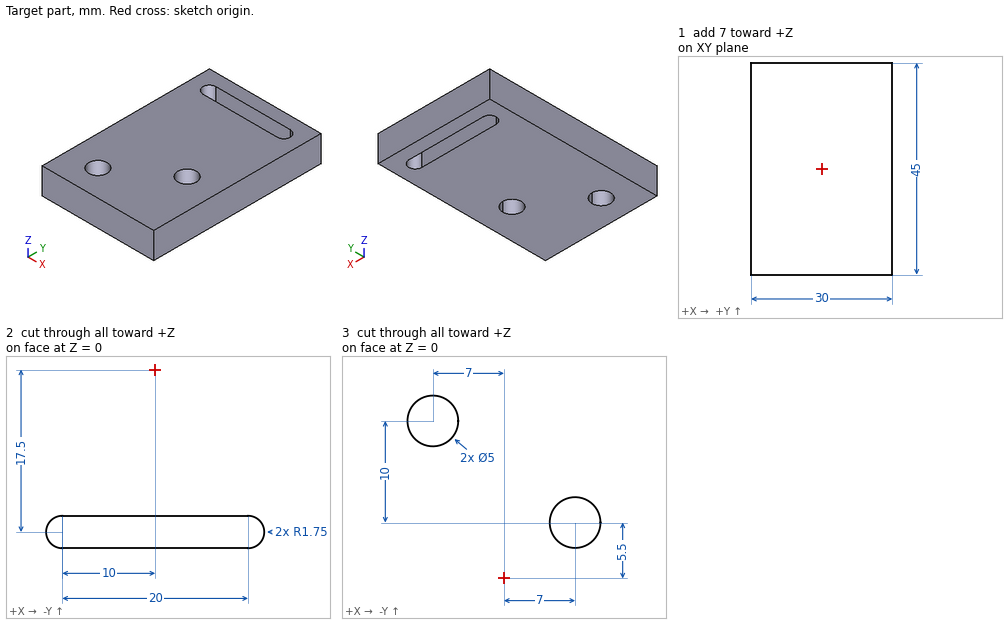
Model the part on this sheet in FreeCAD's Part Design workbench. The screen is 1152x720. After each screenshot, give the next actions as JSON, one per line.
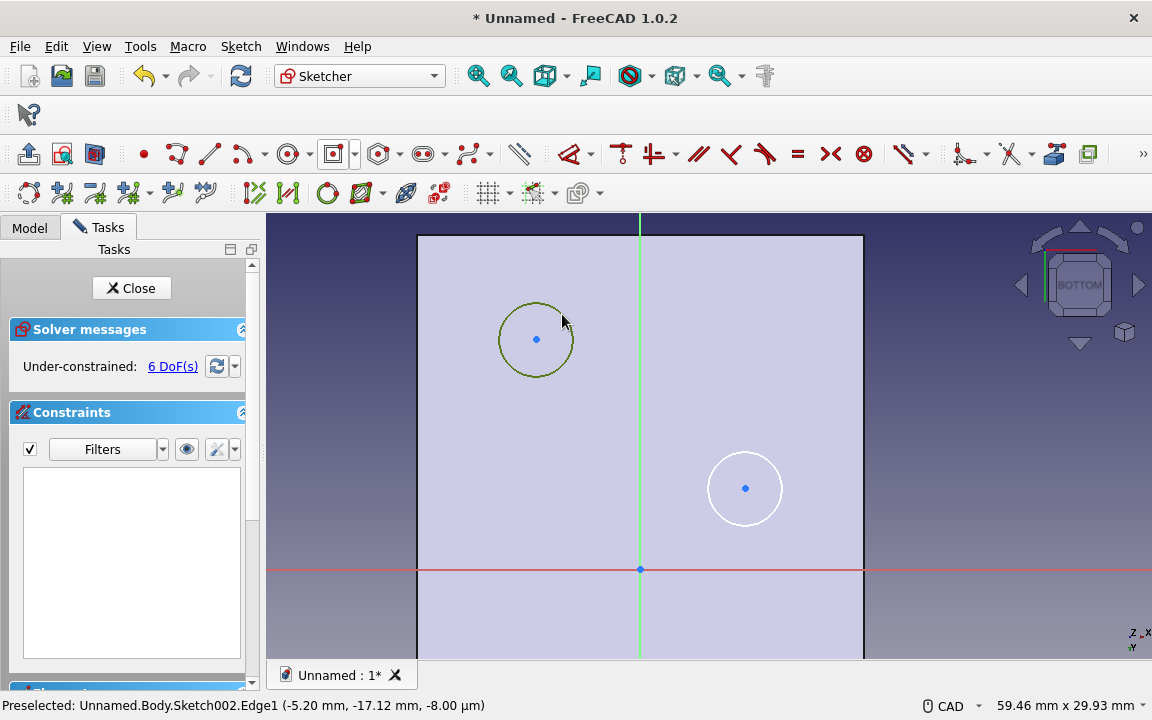
{"action": "left_click", "coordinate": [771, 463]}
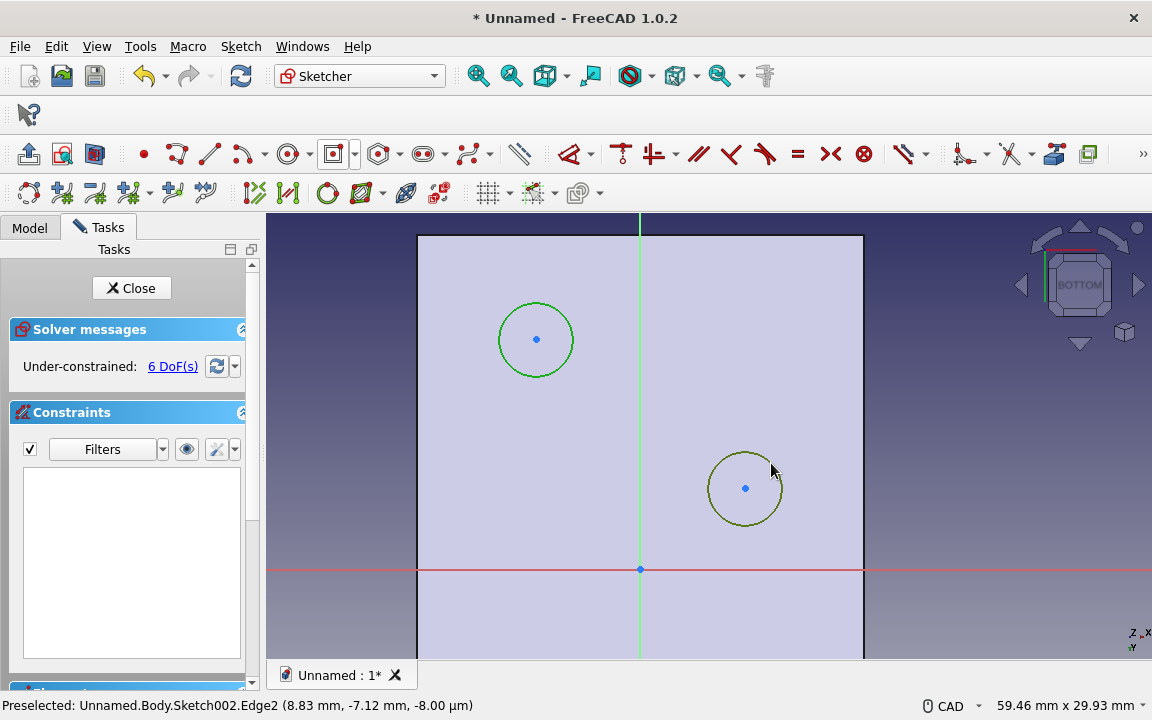
{"action": "left_click", "coordinate": [798, 154]}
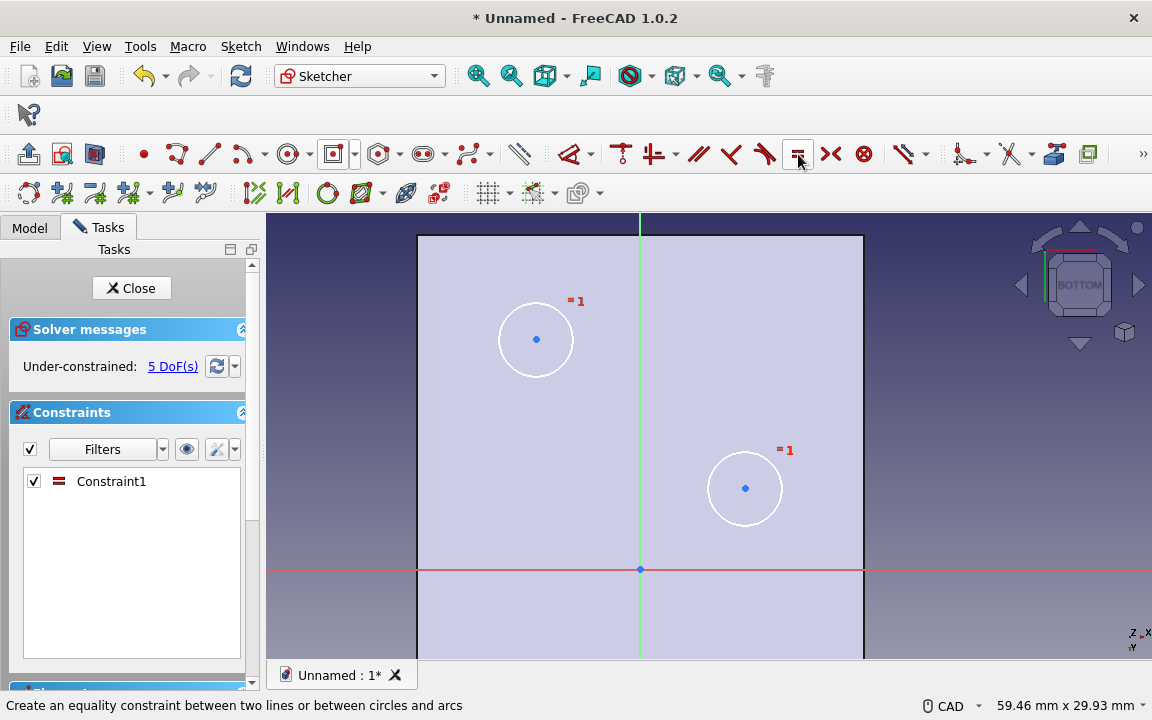
{"action": "left_click", "coordinate": [568, 154]}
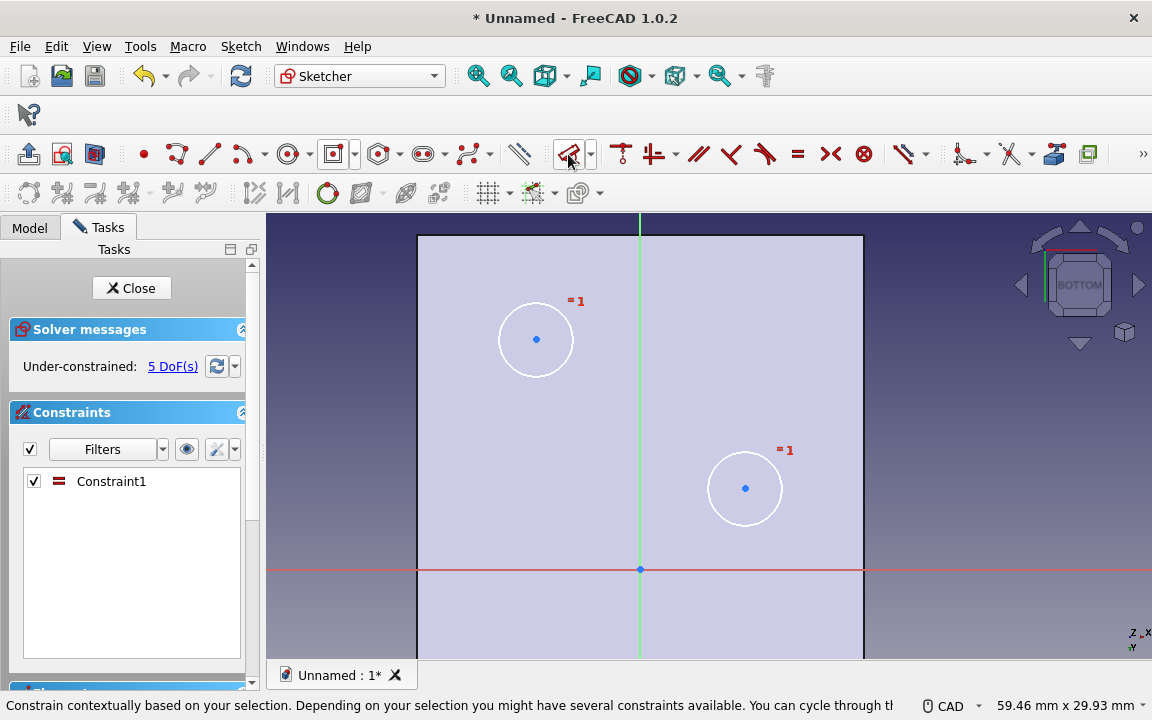
{"action": "left_click", "coordinate": [562, 314]}
{"action": "left_click", "coordinate": [585, 291]}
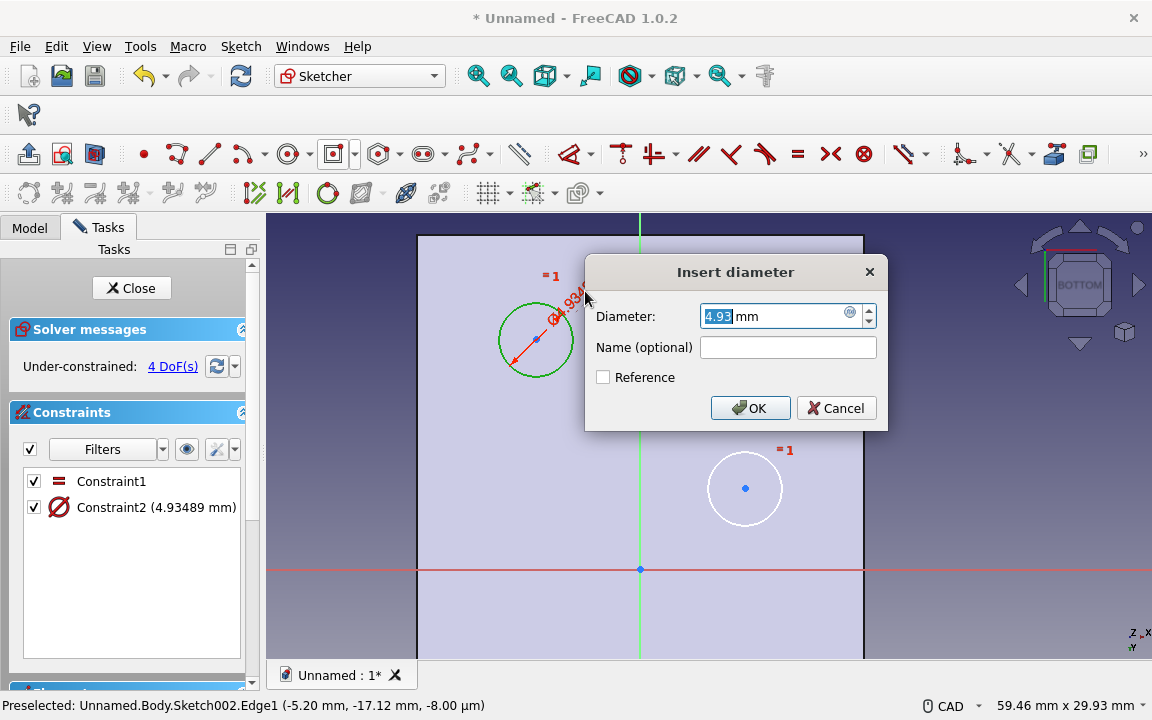
{"action": "type", "text": "5"}
{"action": "key", "text": "Return"}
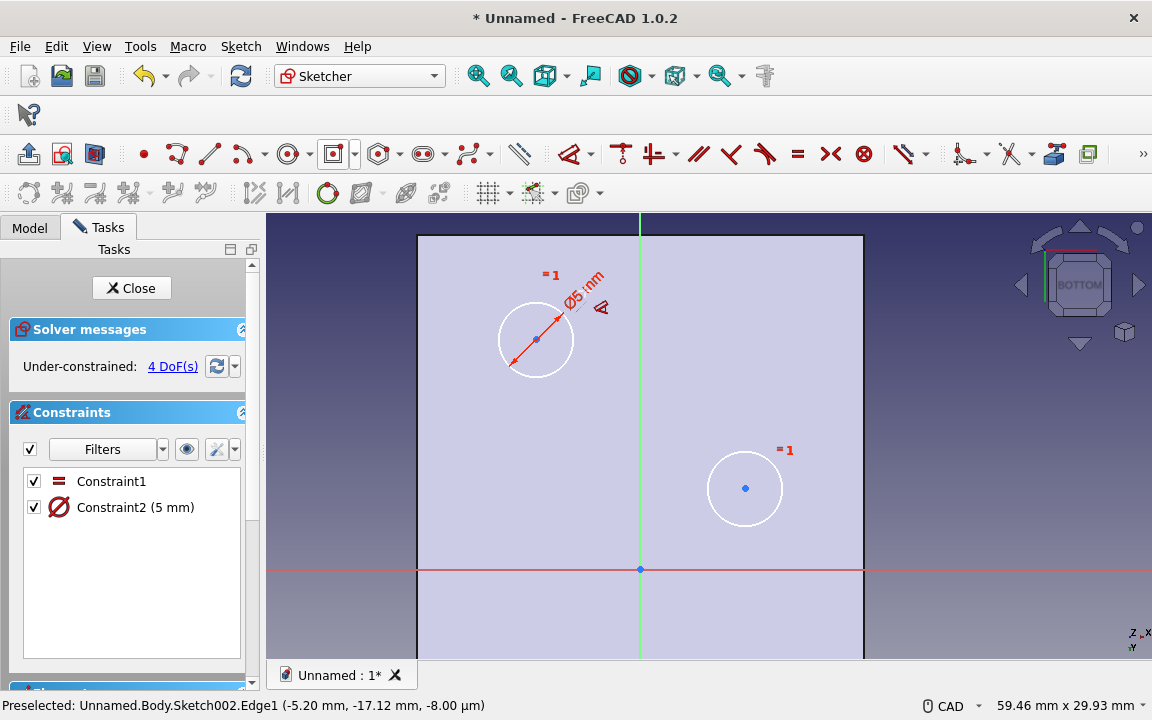
{"action": "left_click", "coordinate": [536, 340]}
{"action": "left_click", "coordinate": [588, 604]}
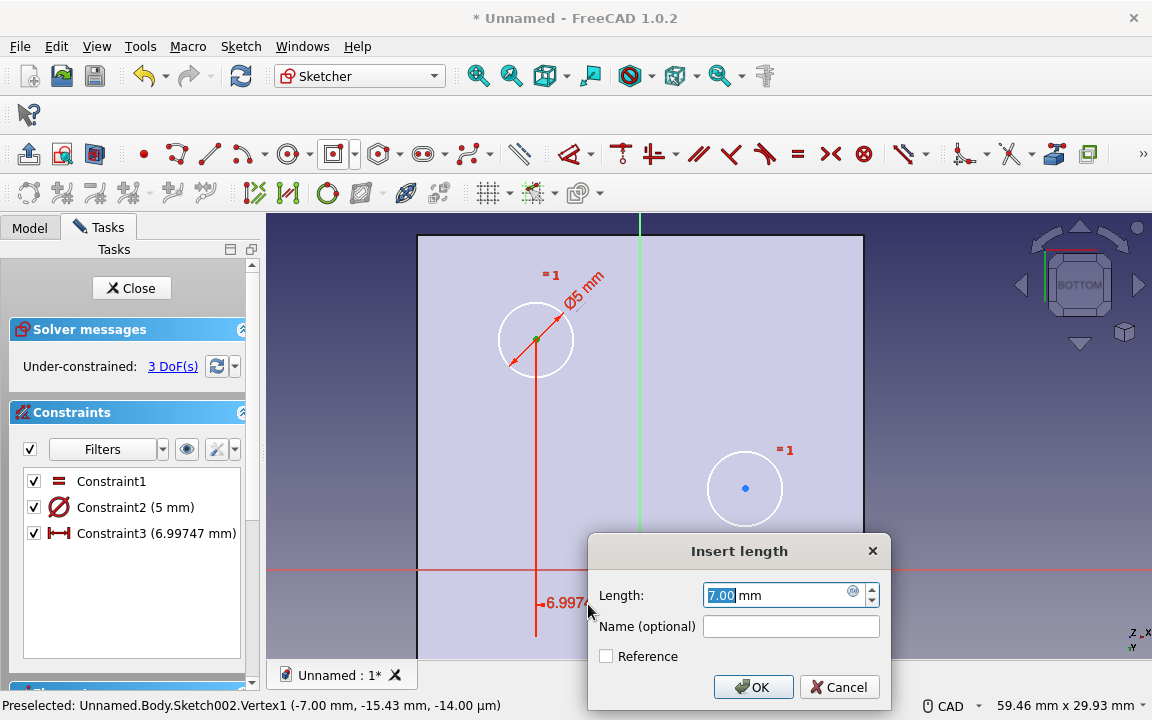
{"action": "type", "text": "7"}
{"action": "key", "text": "Return"}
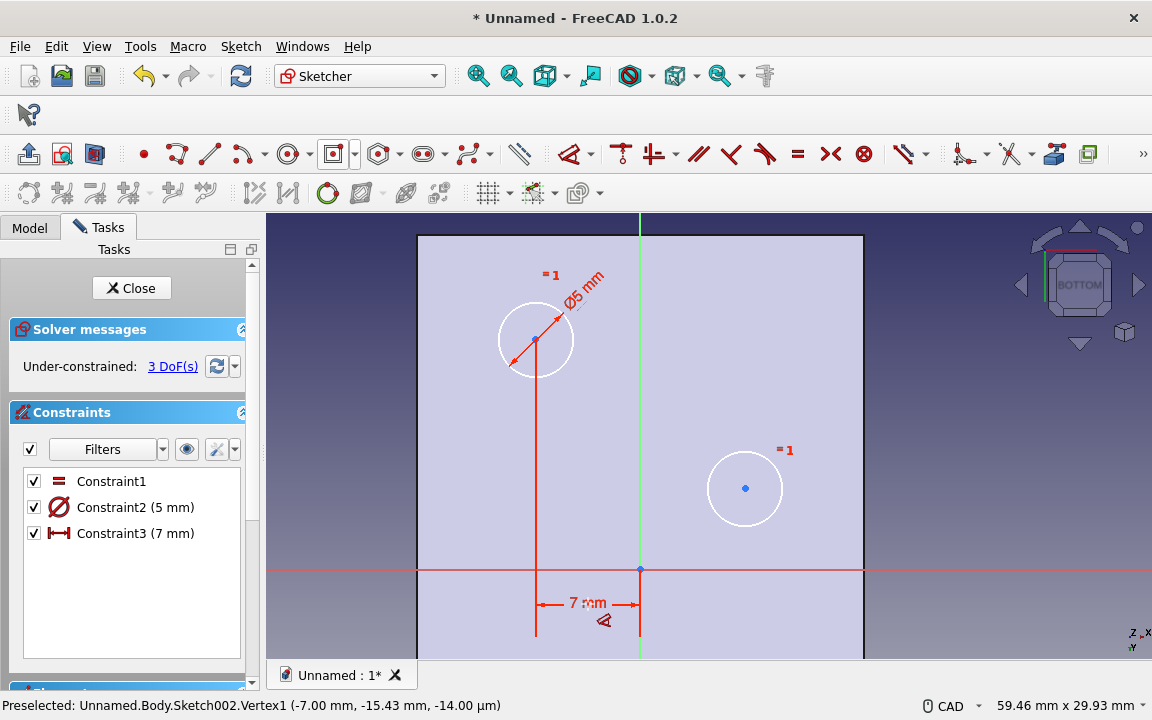
{"action": "left_click", "coordinate": [745, 489]}
{"action": "left_click", "coordinate": [693, 604]}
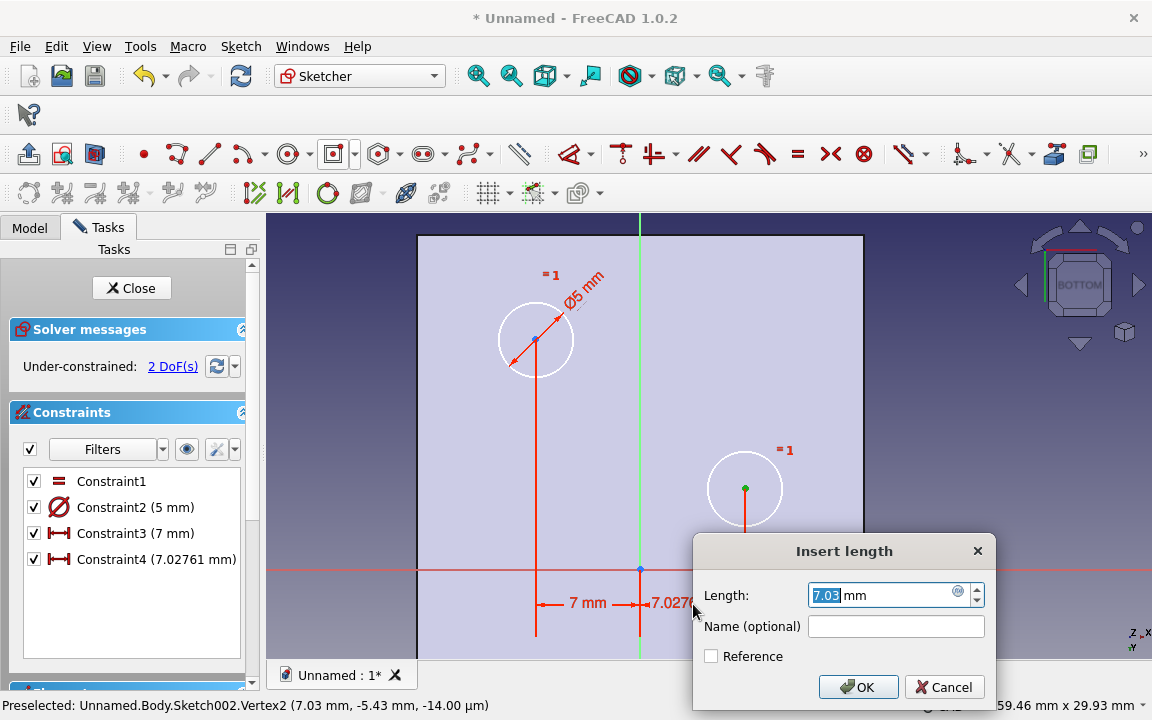
{"action": "type", "text": "7"}
{"action": "key", "text": "Return"}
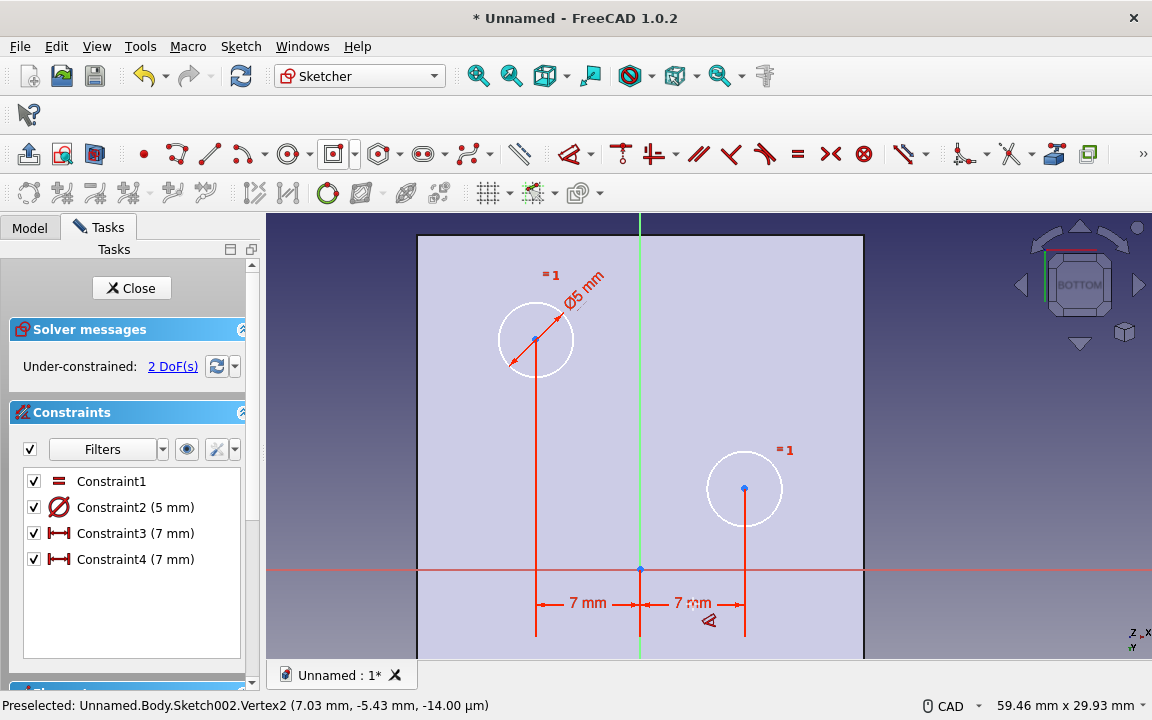
{"action": "left_click", "coordinate": [745, 489]}
{"action": "left_click", "coordinate": [779, 529]}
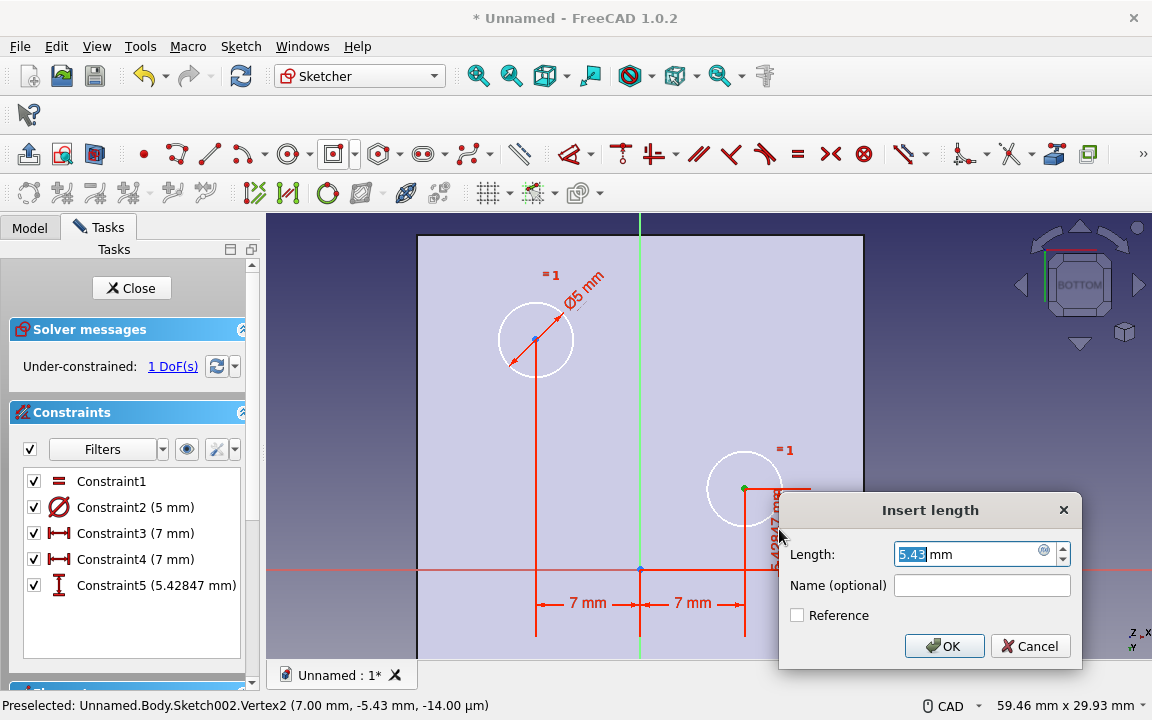
{"action": "type", "text": "5.5"}
{"action": "key", "text": "Return"}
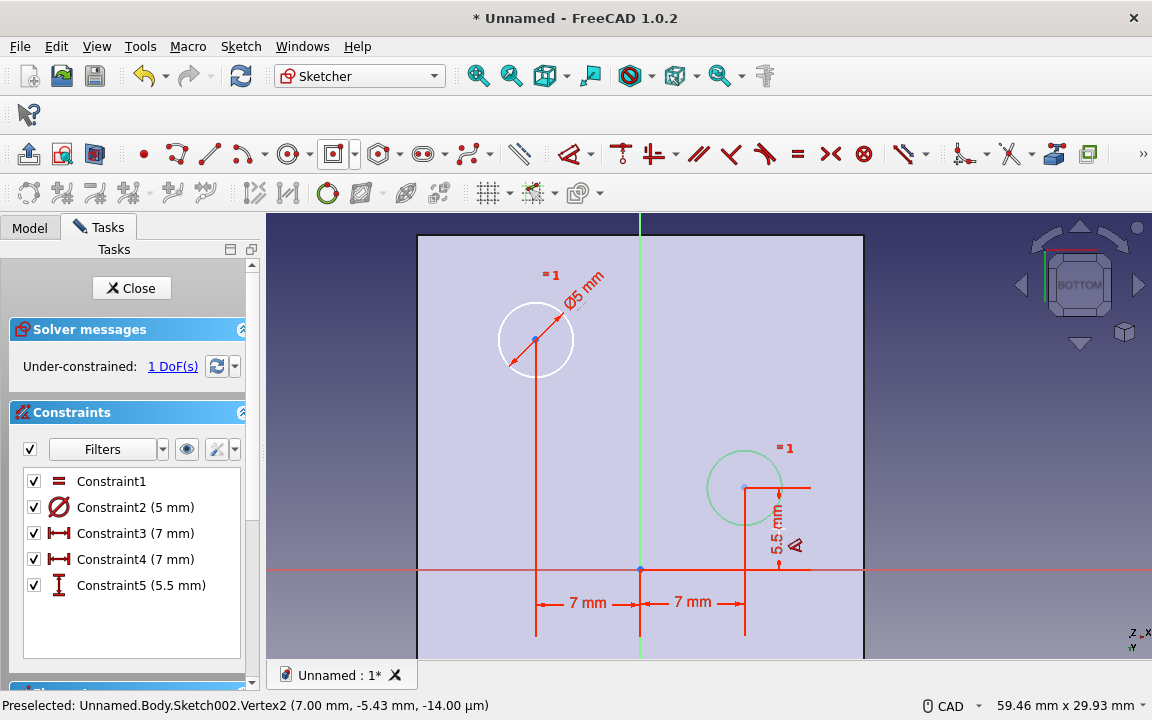
{"action": "left_click", "coordinate": [536, 340]}